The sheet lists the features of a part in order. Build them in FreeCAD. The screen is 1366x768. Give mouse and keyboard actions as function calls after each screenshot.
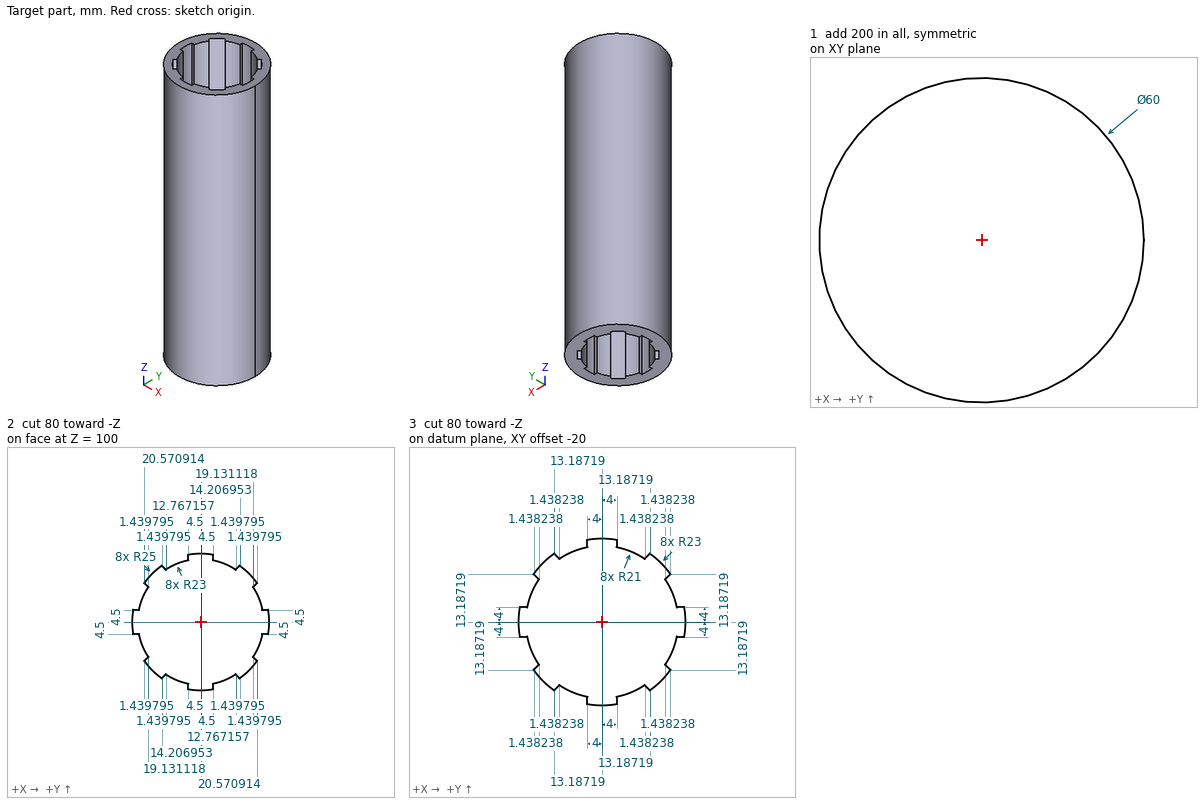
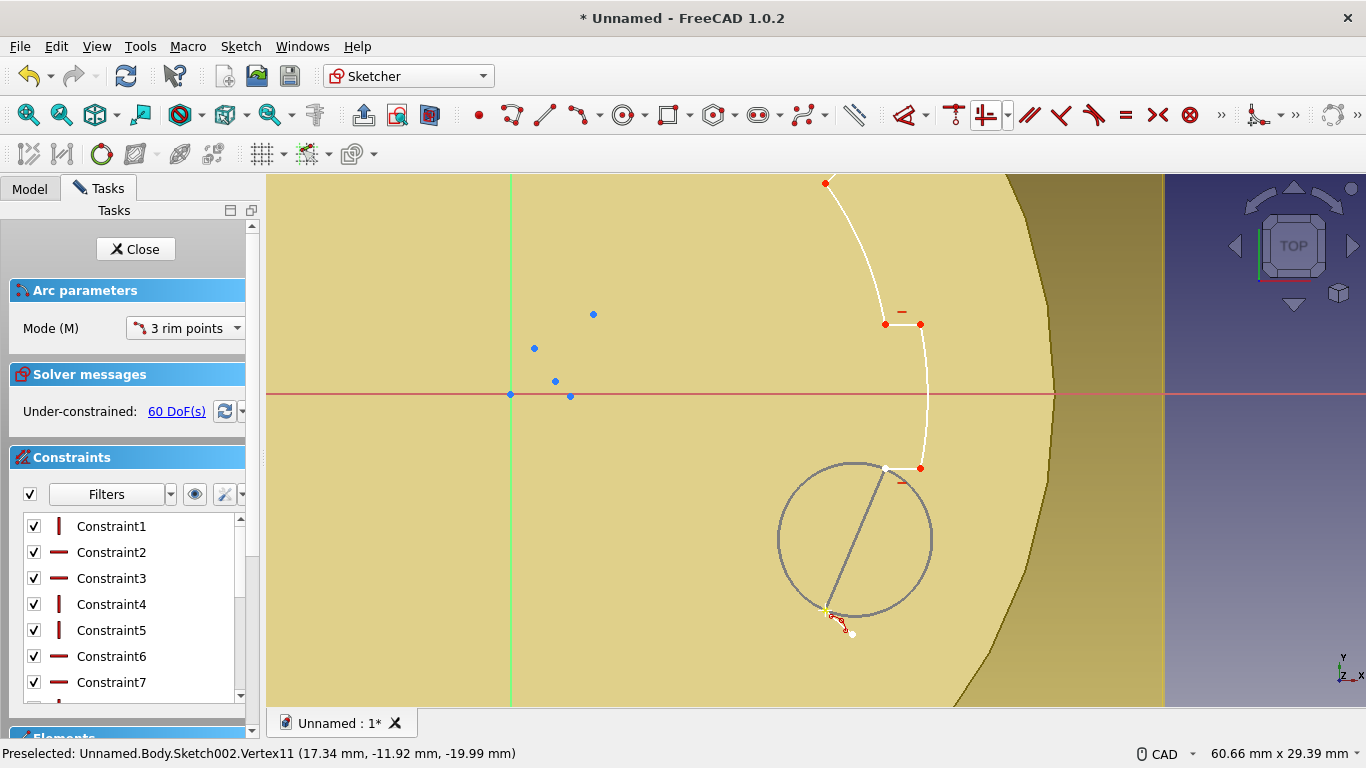
scroll(863, 540, up, 4)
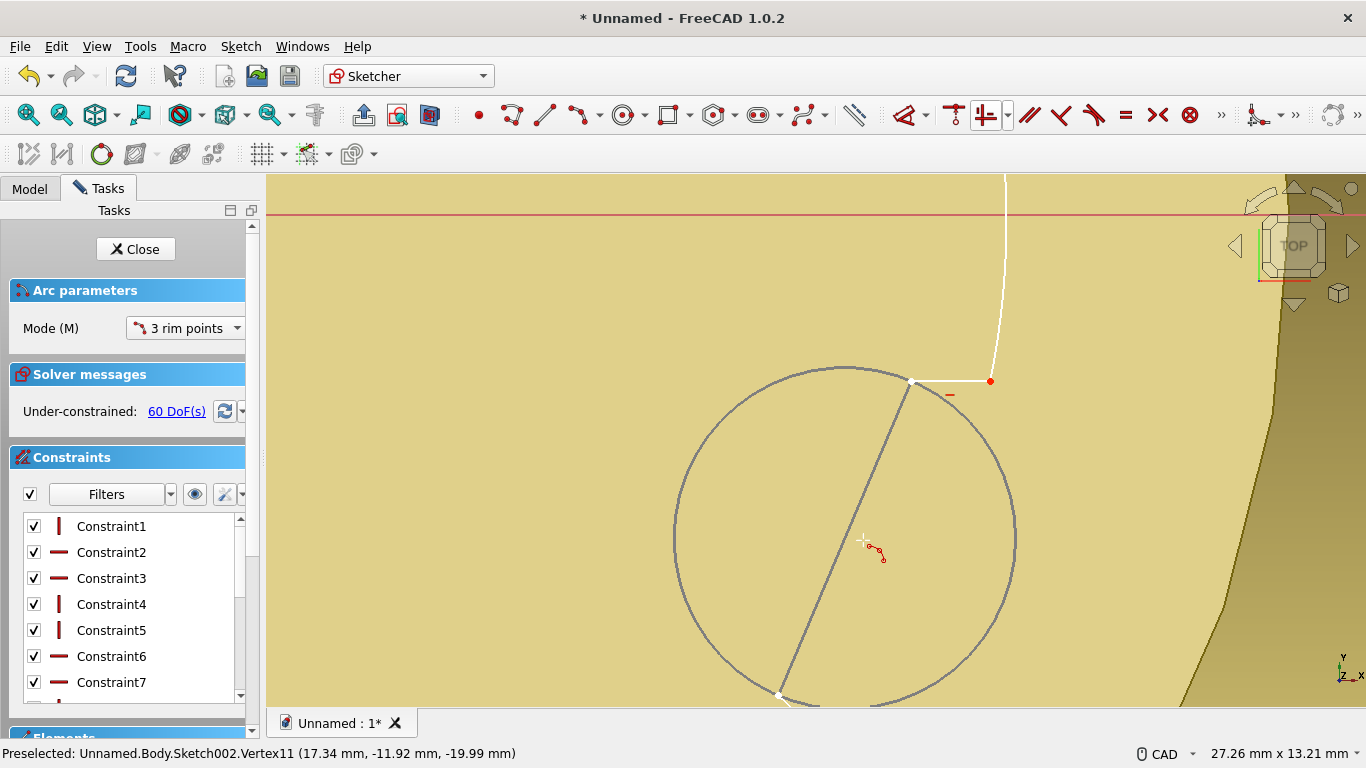
click(862, 539)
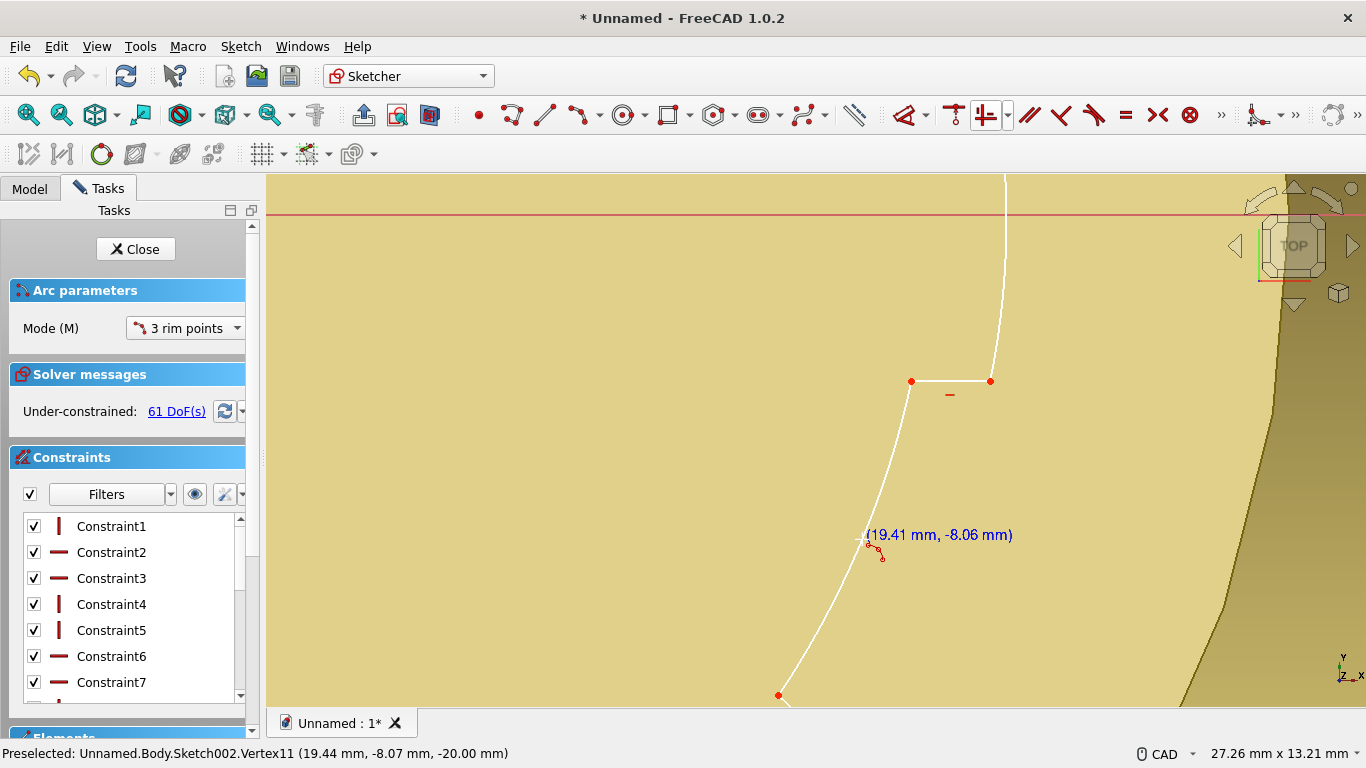
scroll(880, 485, down, 9)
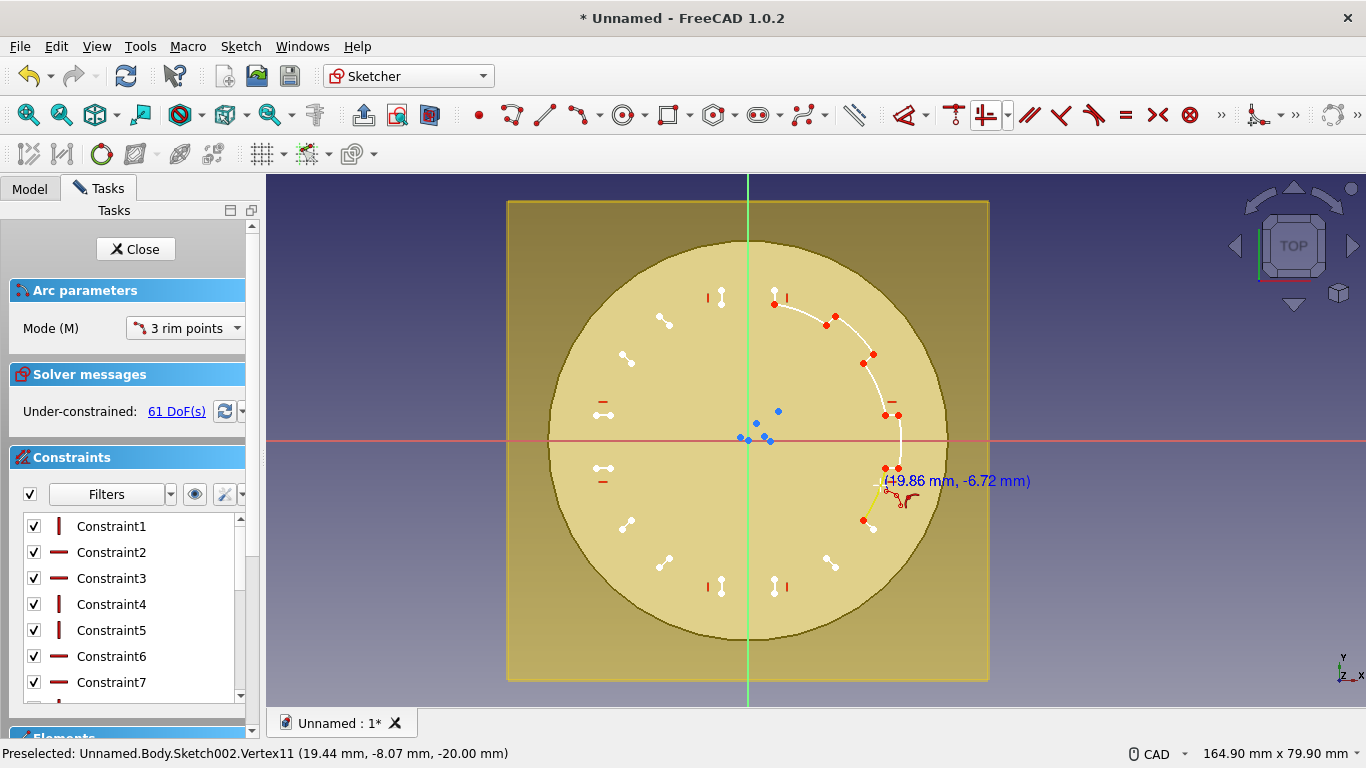
scroll(874, 529, up, 5)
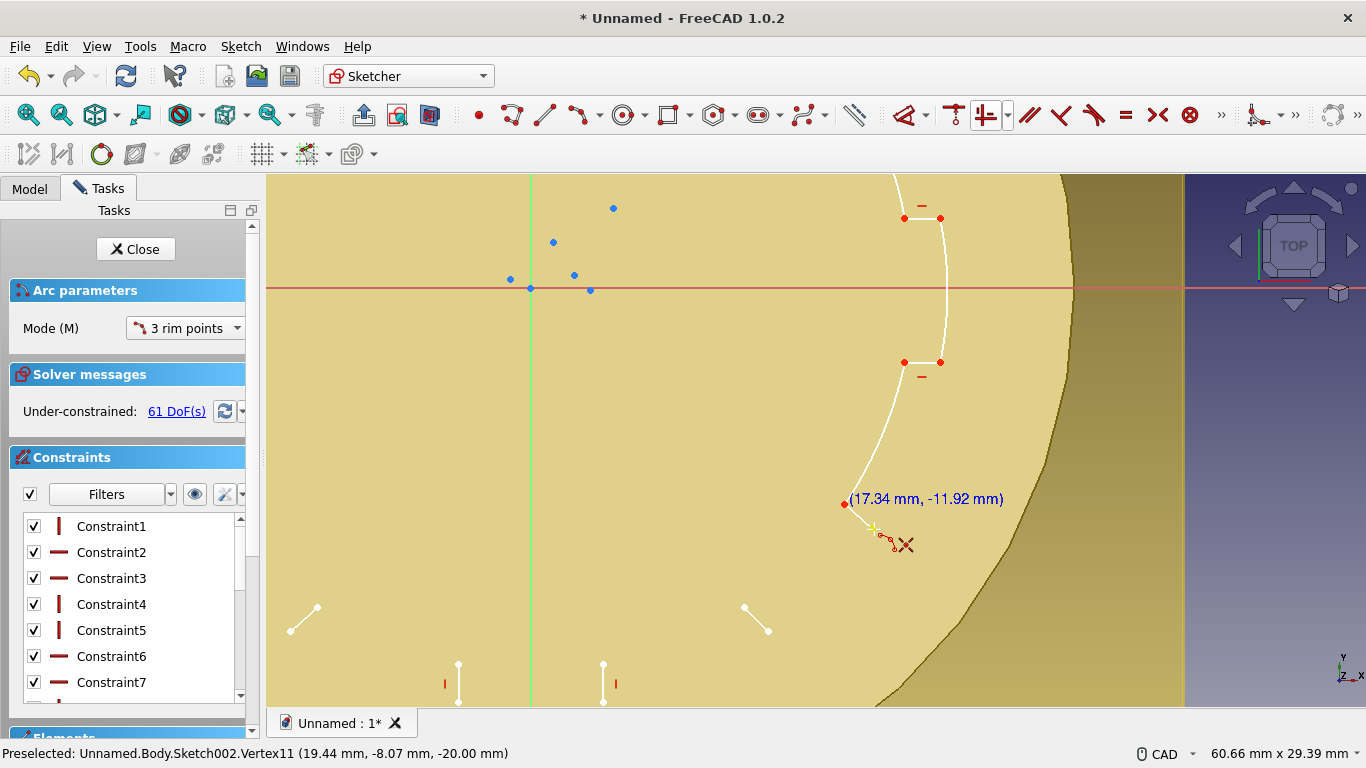
click(872, 529)
click(769, 632)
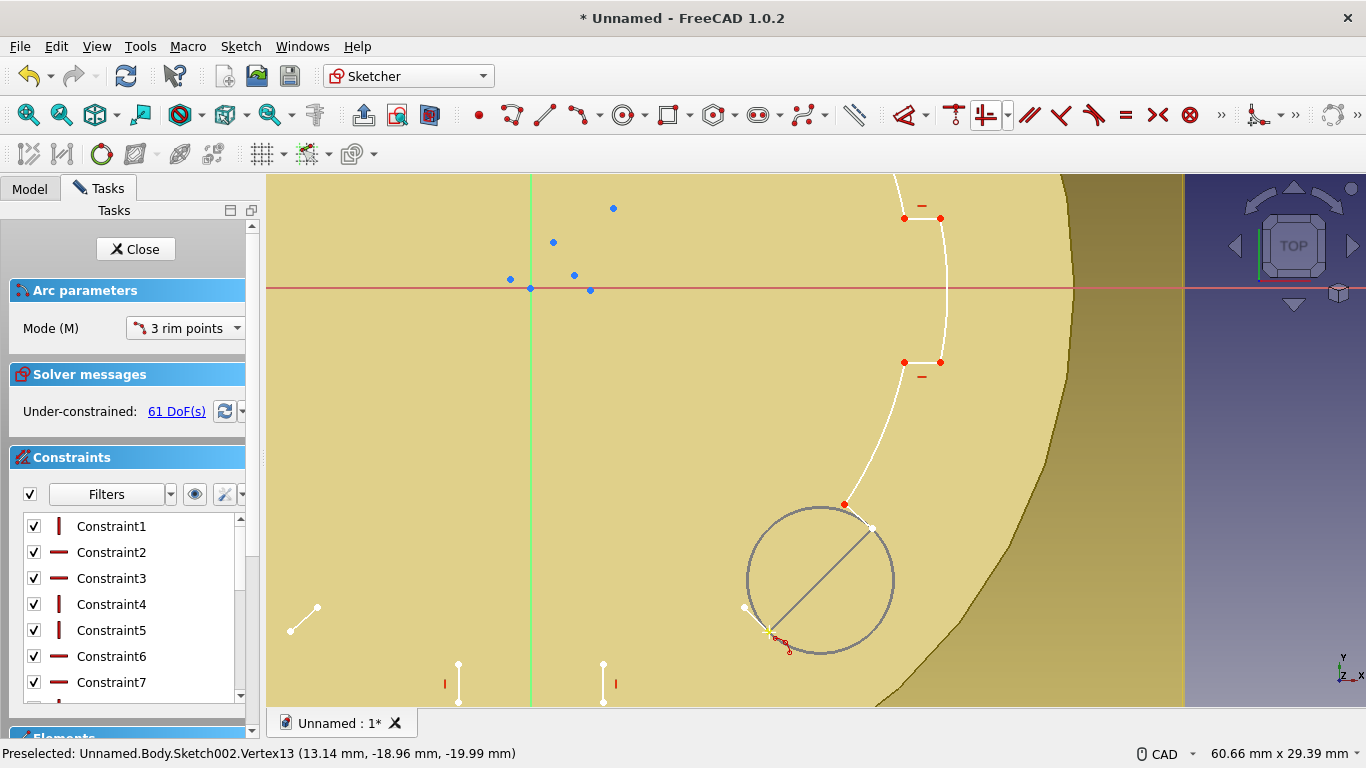
scroll(825, 583, up, 5)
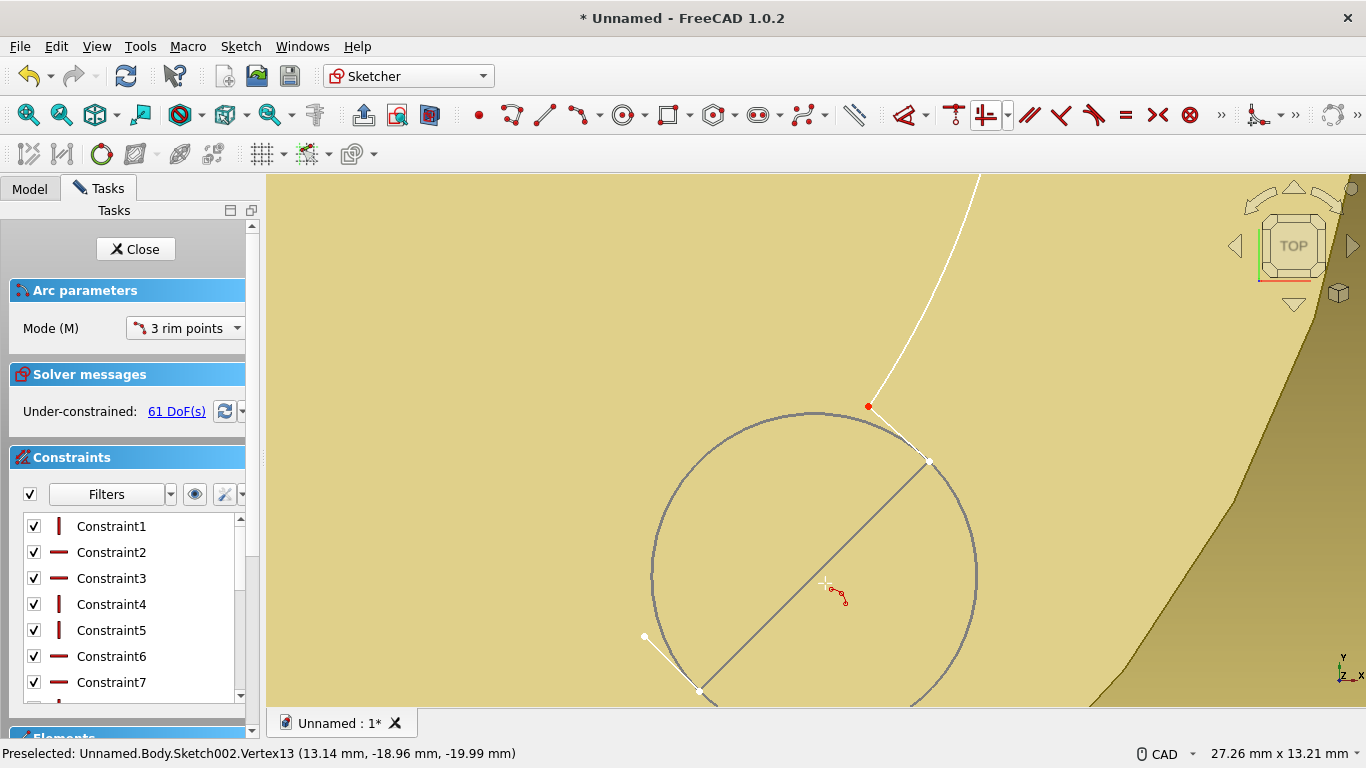
click(825, 582)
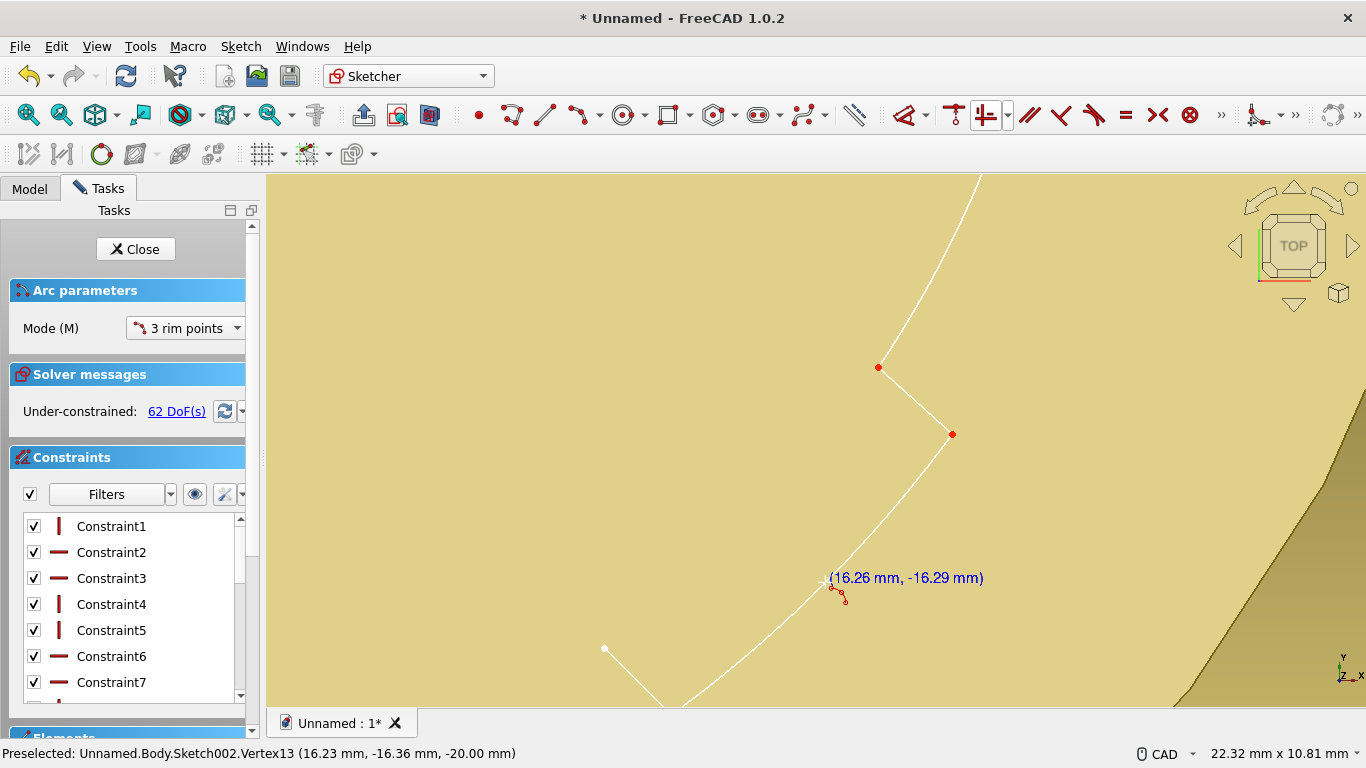
scroll(861, 544, down, 10)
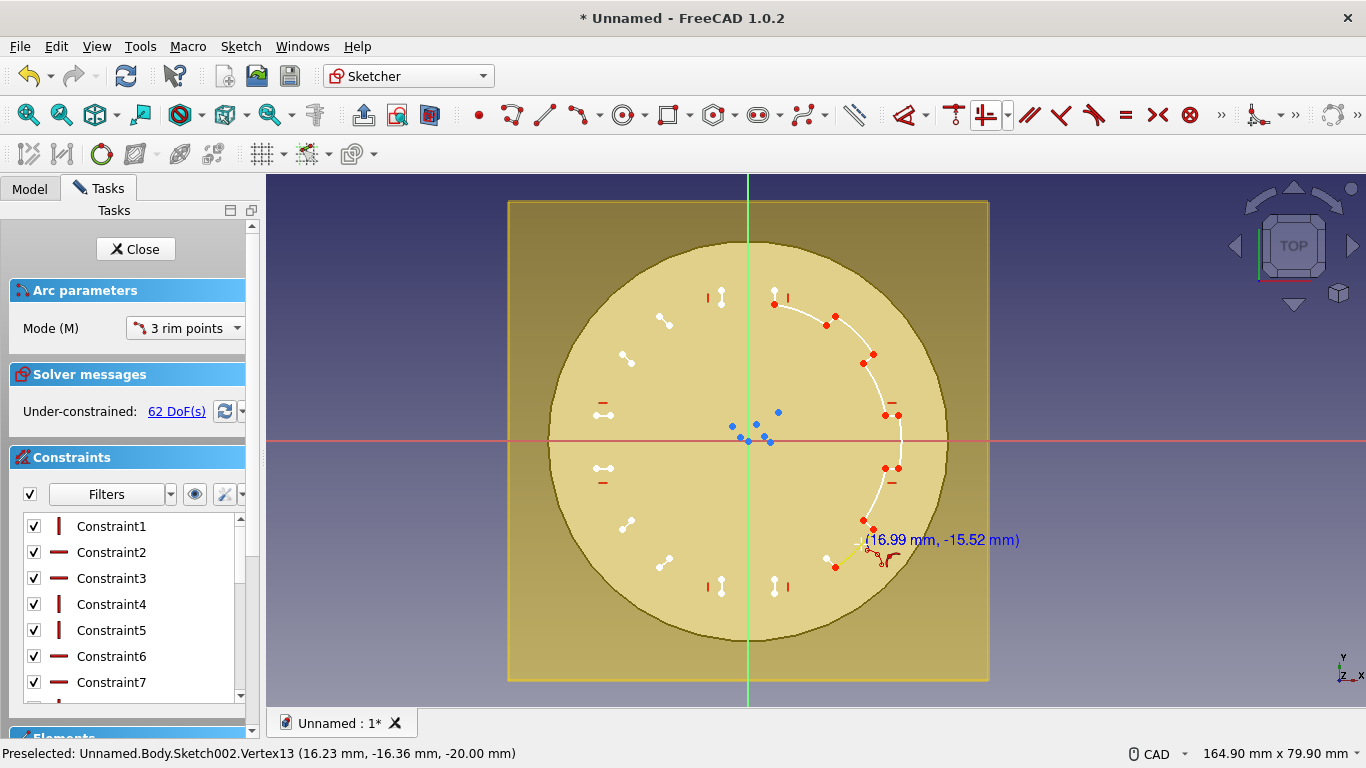
scroll(827, 557, up, 5)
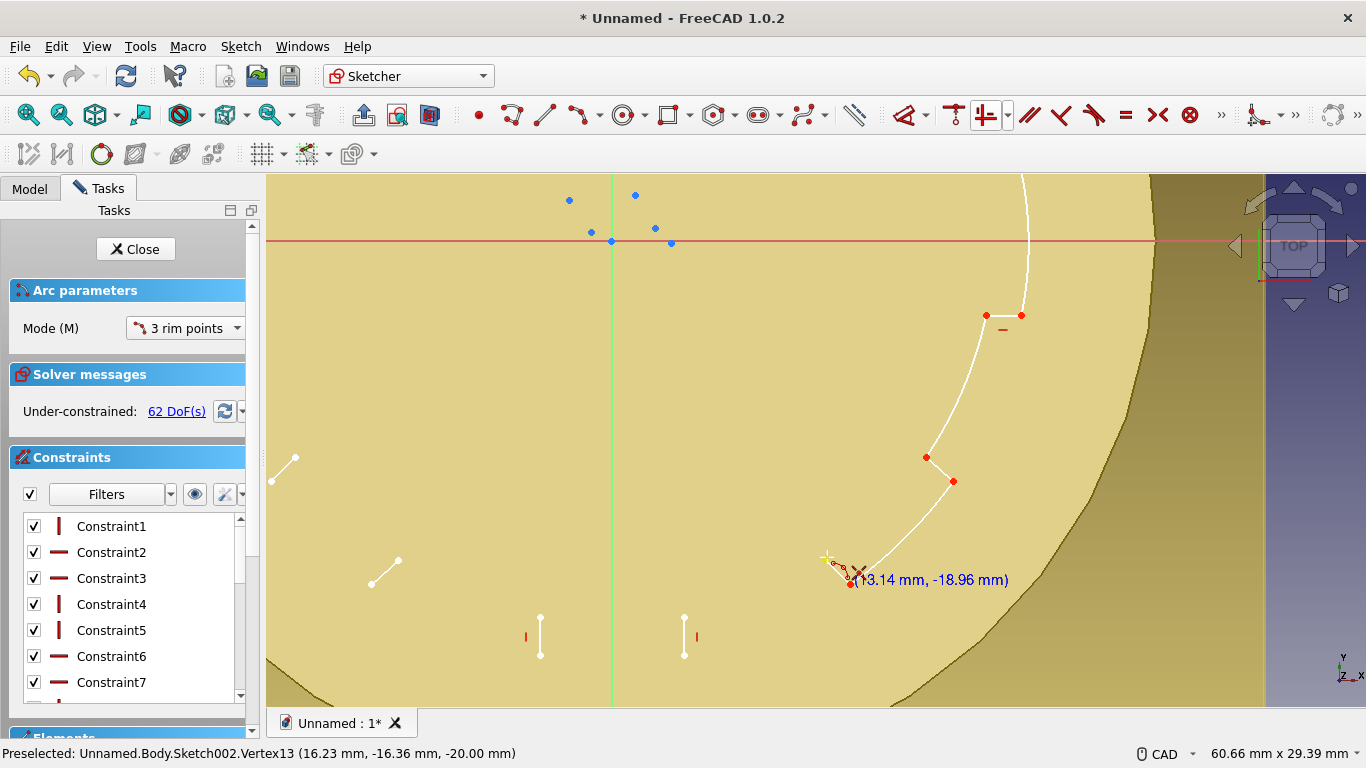
click(826, 560)
click(684, 618)